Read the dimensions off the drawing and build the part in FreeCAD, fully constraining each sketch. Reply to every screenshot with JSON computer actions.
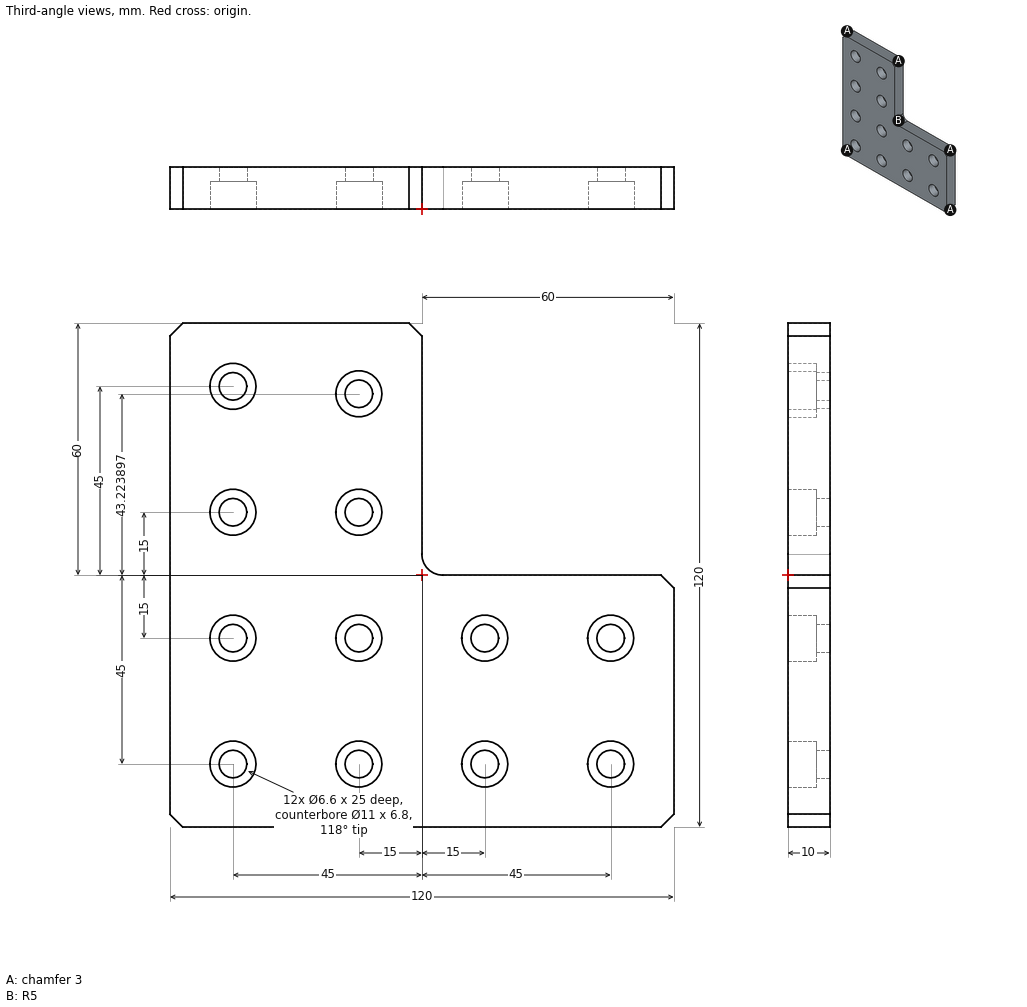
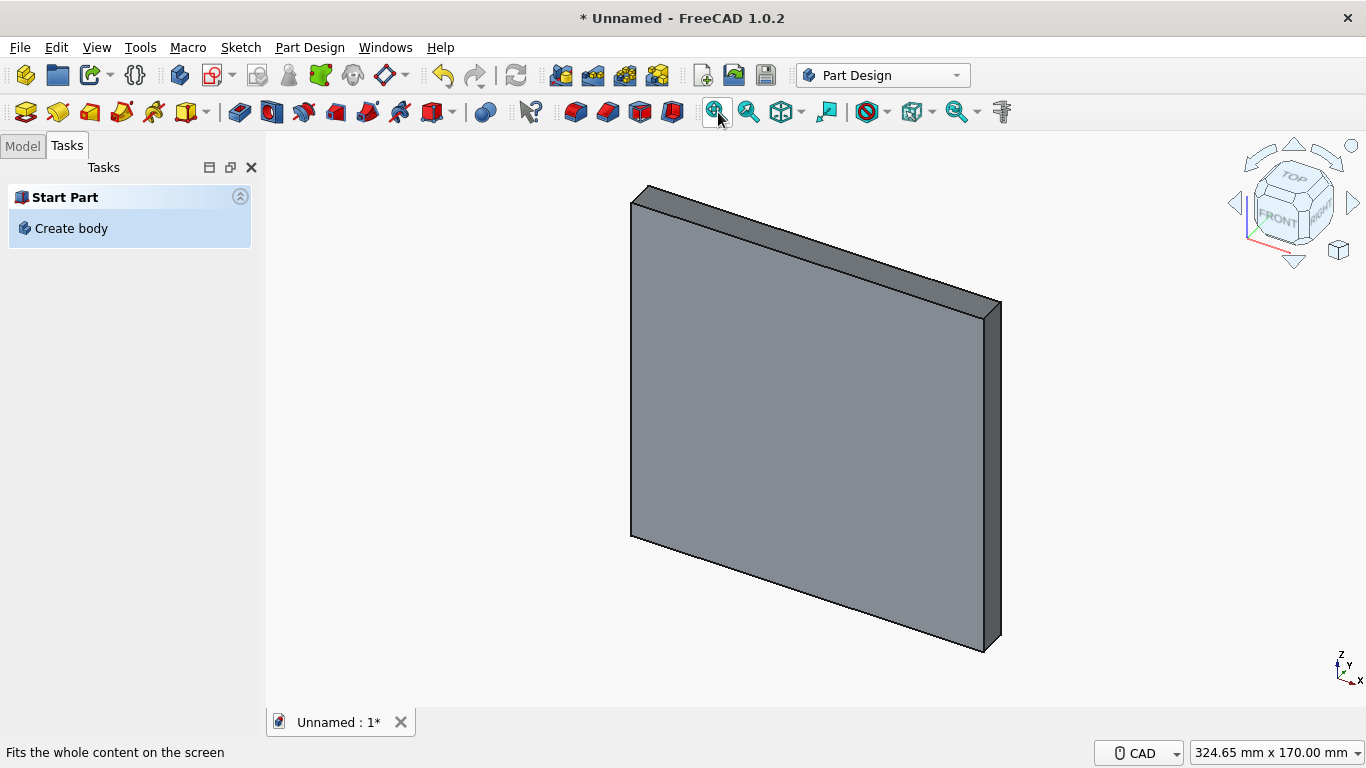
{"action": "key", "text": "4"}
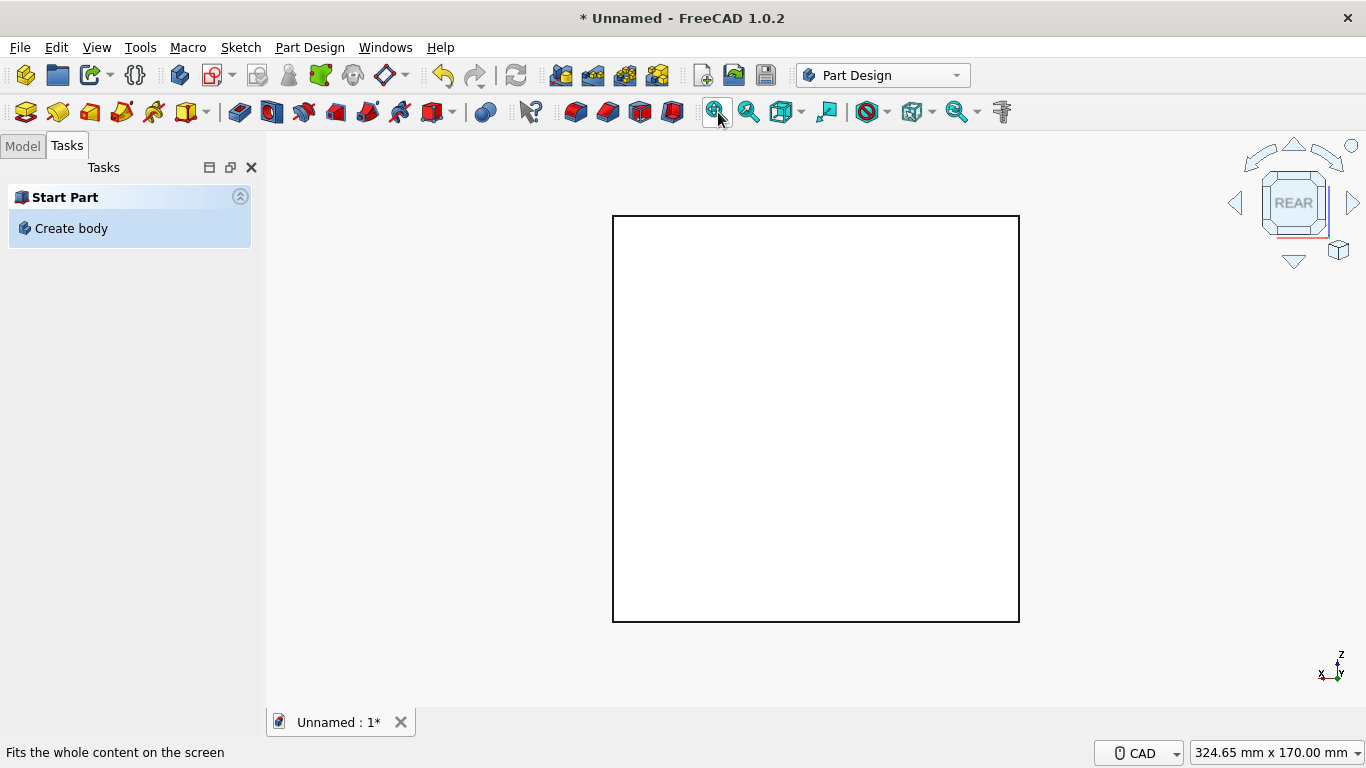
{"action": "left_click", "coordinate": [816, 418]}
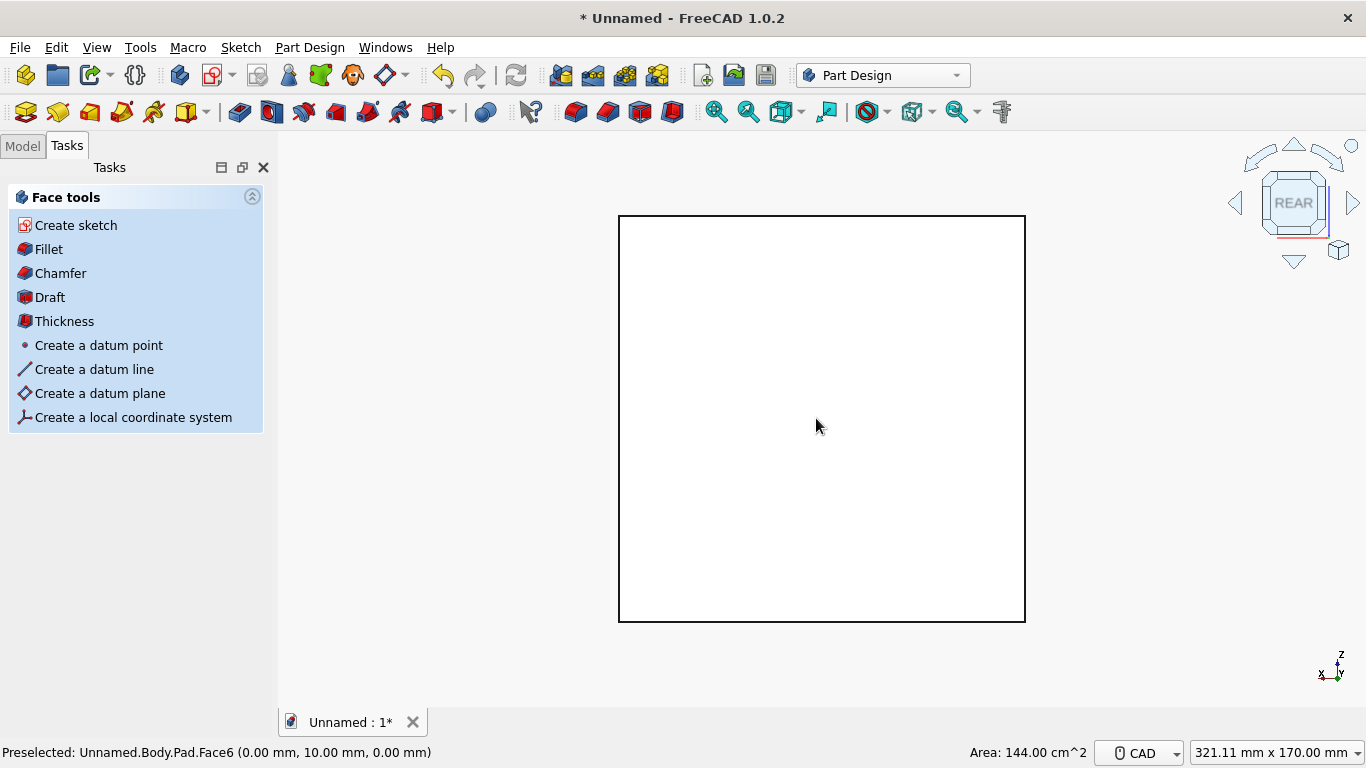
{"action": "left_click", "coordinate": [212, 76]}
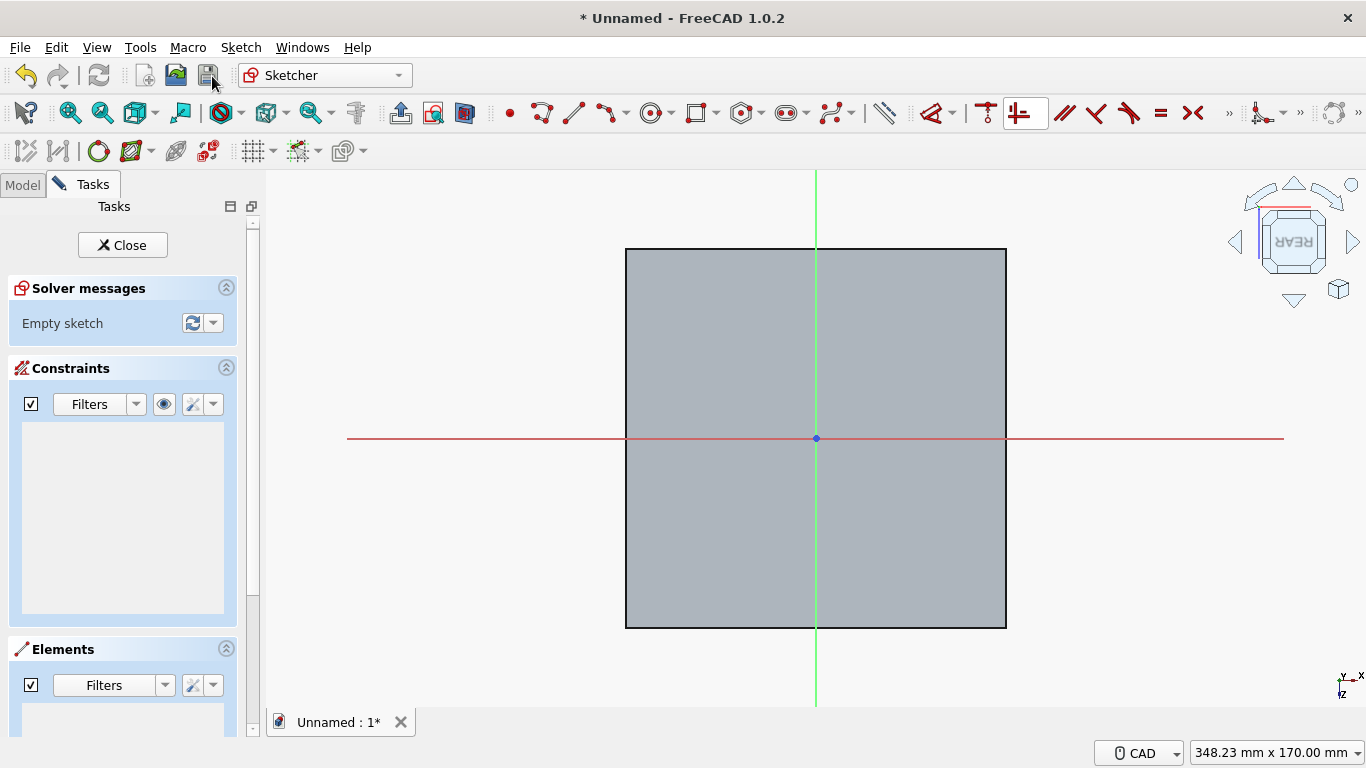
{"action": "scroll", "coordinate": [1109, 649], "scroll_direction": "up", "scroll_amount": 3}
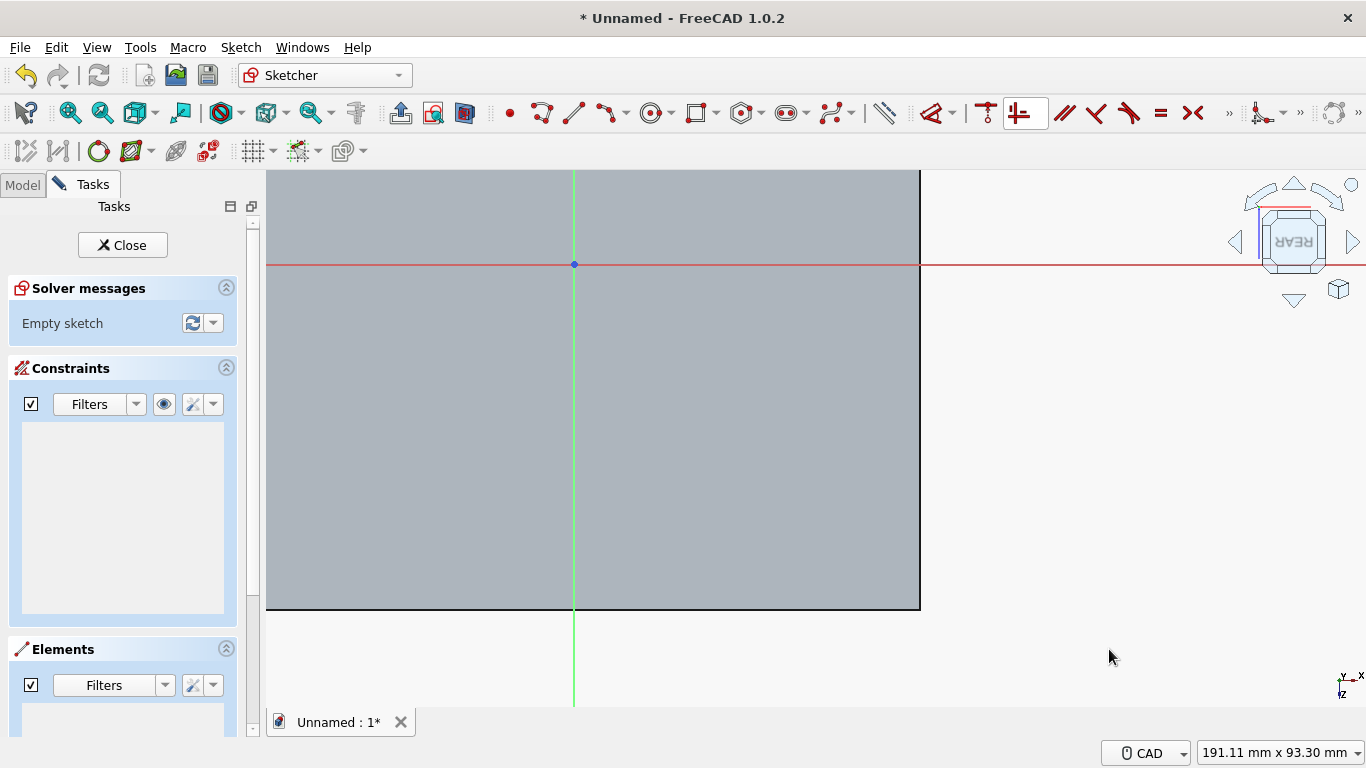
{"action": "left_click", "coordinate": [696, 114]}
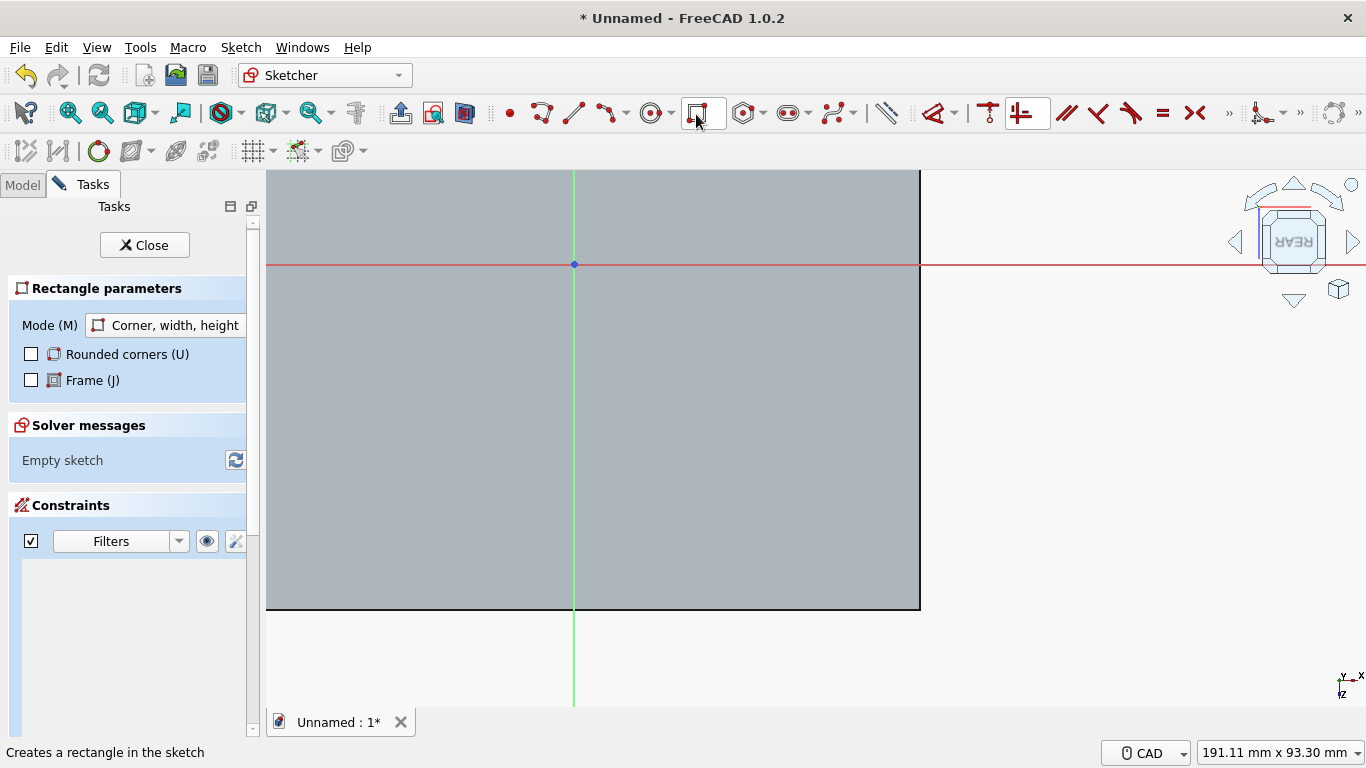
{"action": "left_click", "coordinate": [574, 265]}
{"action": "left_click", "coordinate": [920, 610]}
{"action": "key", "text": "Escape"}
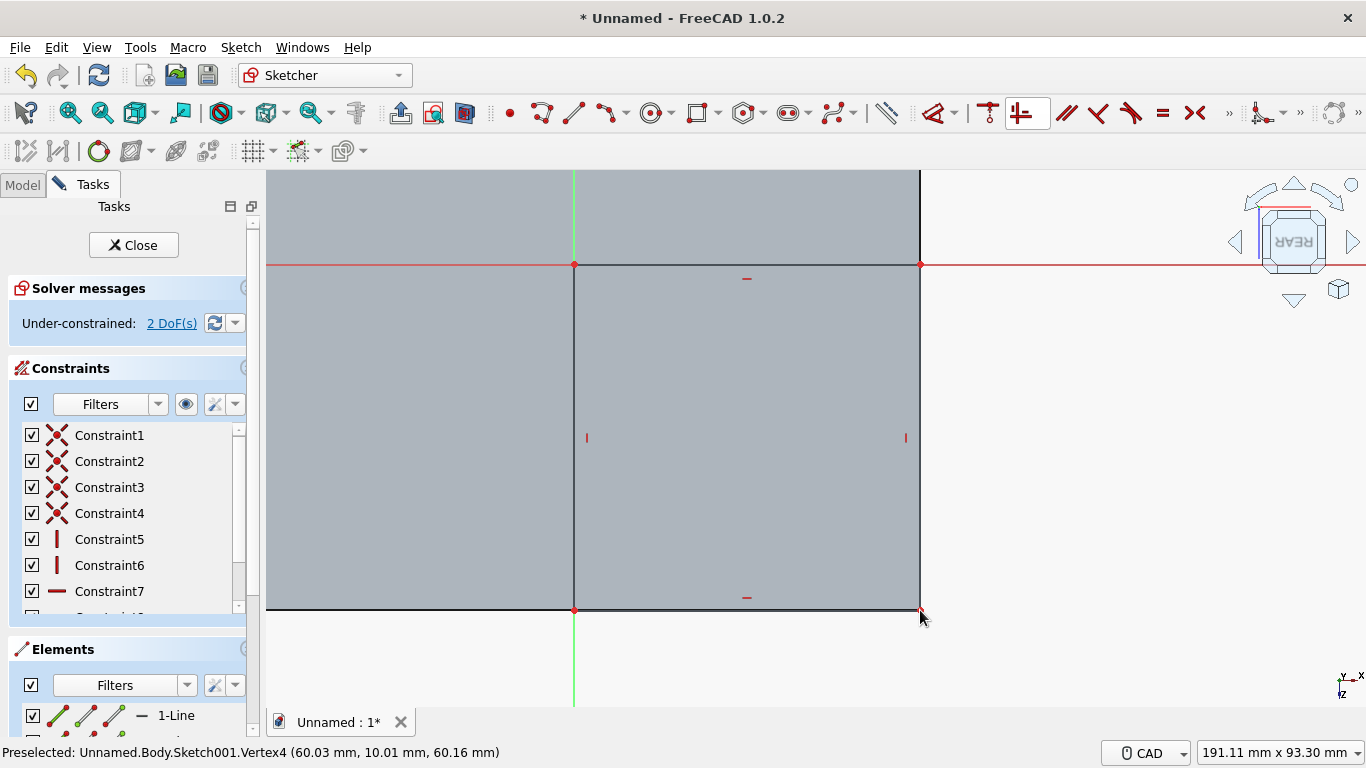
{"action": "left_click", "coordinate": [934, 114]}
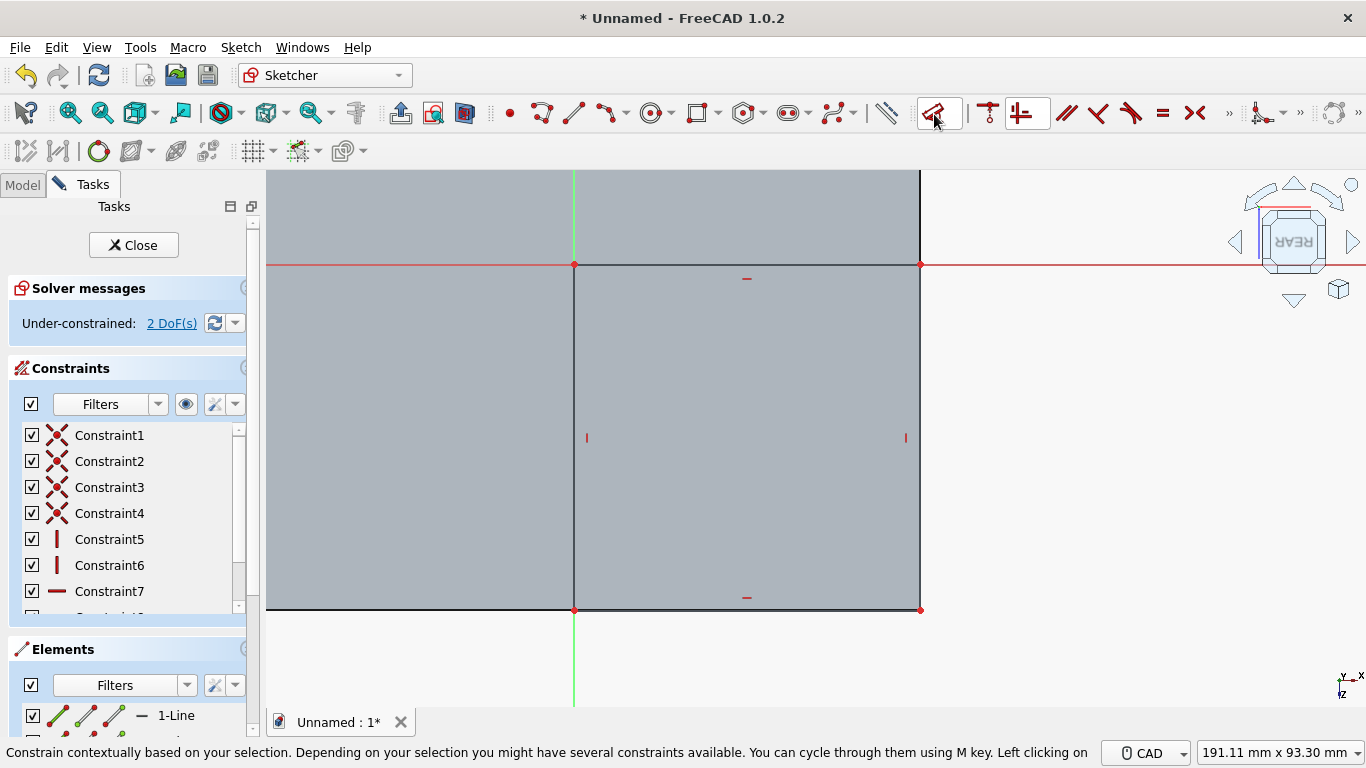
{"action": "left_click", "coordinate": [574, 369]}
{"action": "left_click", "coordinate": [540, 438]}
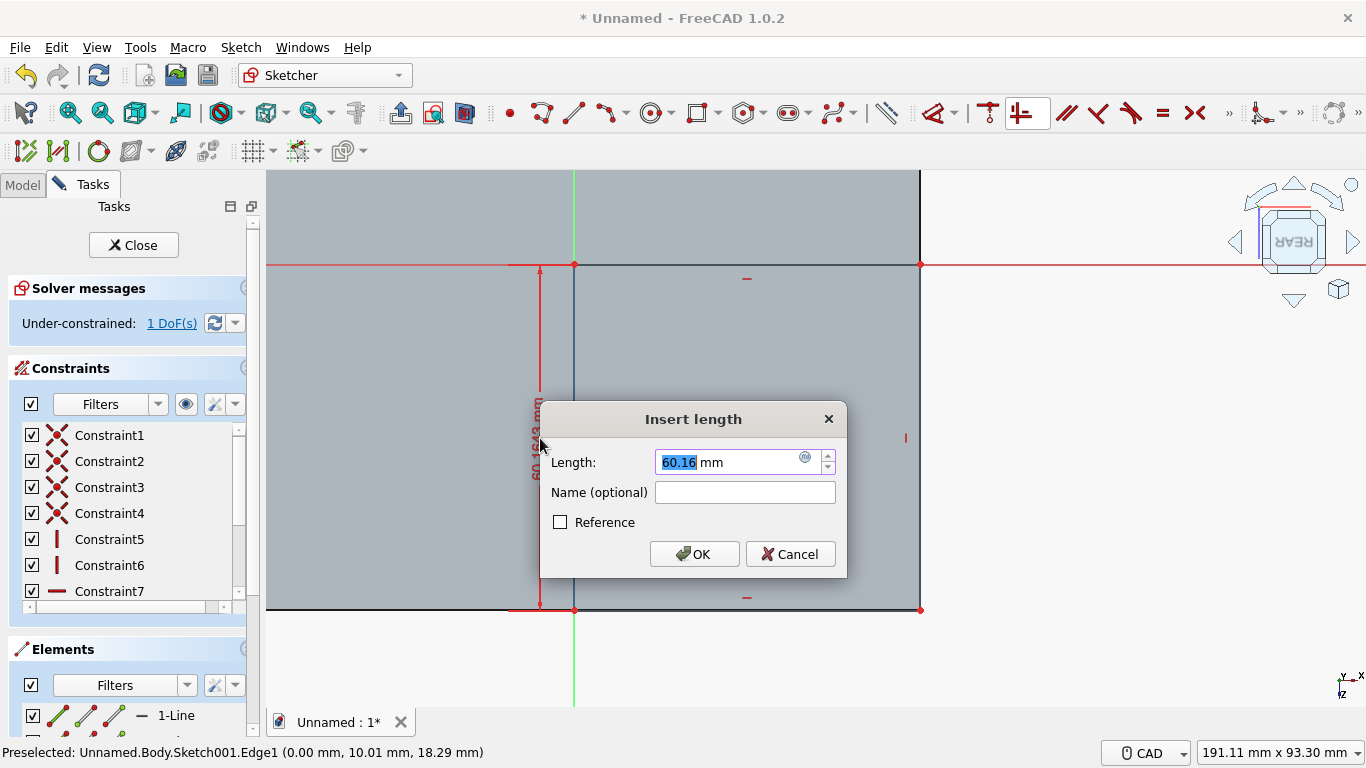
{"action": "type", "text": "60"}
{"action": "key", "text": "Return"}